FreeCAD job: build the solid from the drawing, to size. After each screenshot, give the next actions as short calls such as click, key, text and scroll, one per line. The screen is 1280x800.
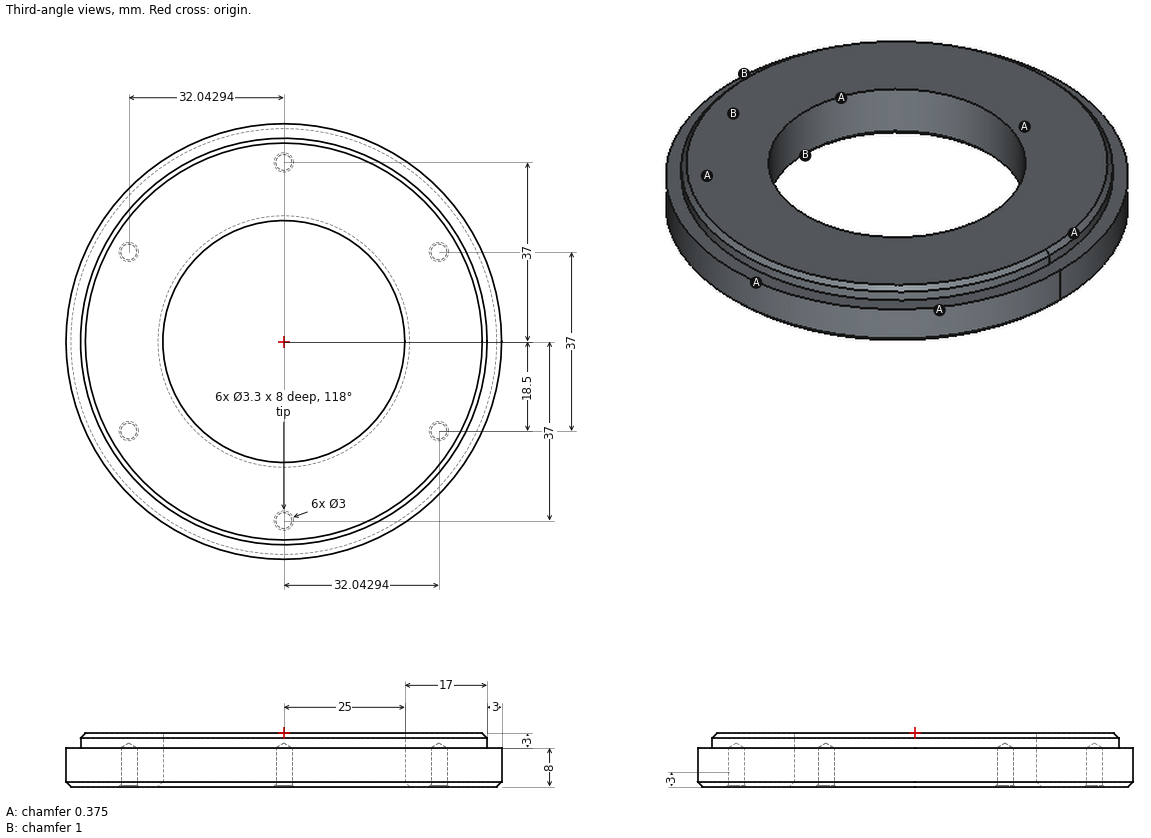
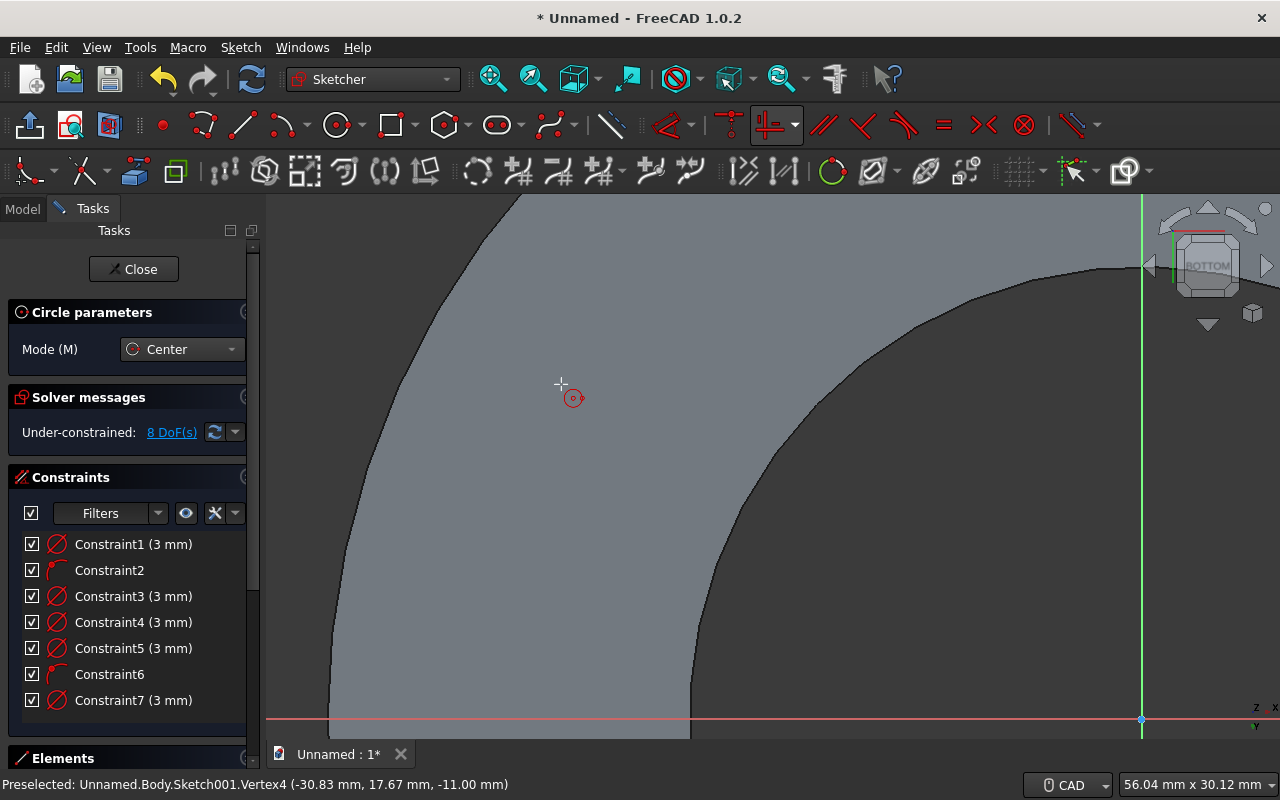
click(562, 385)
move(581, 366)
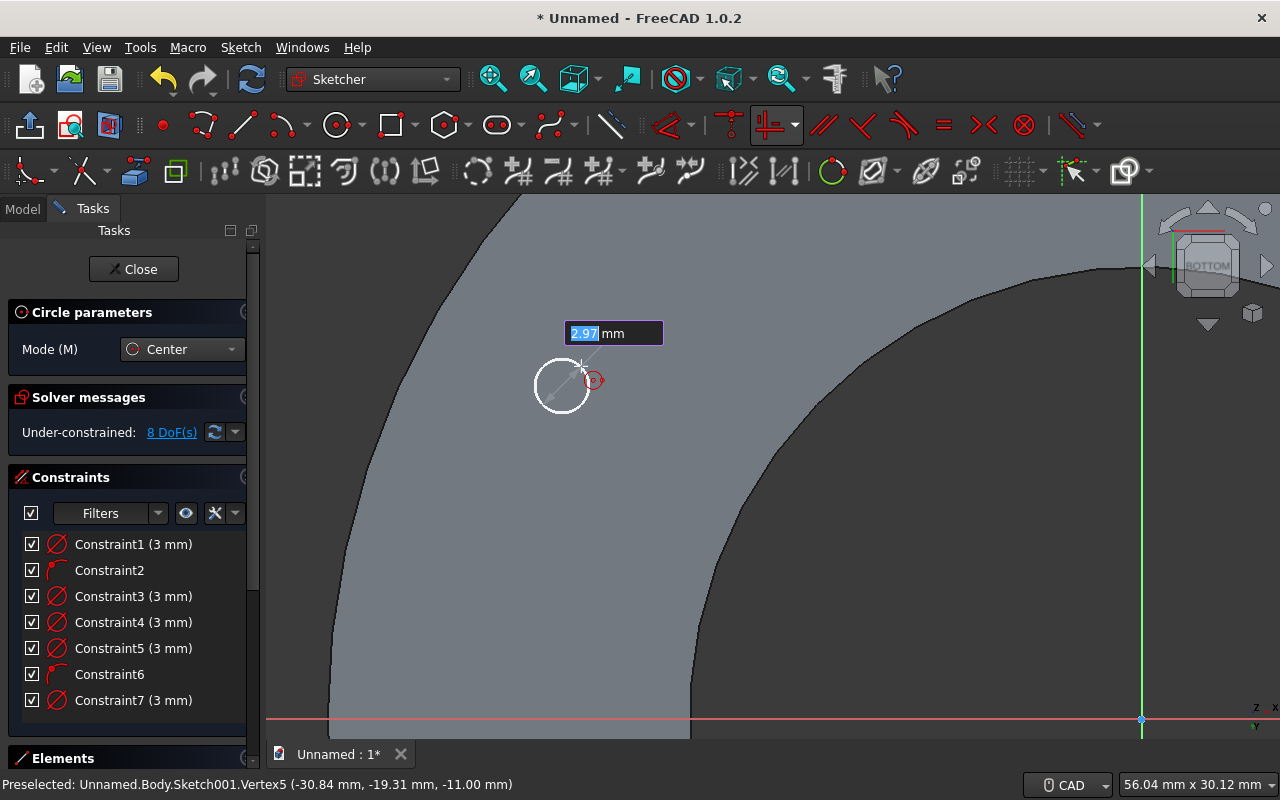
text(3)
key(Return)
key(Escape)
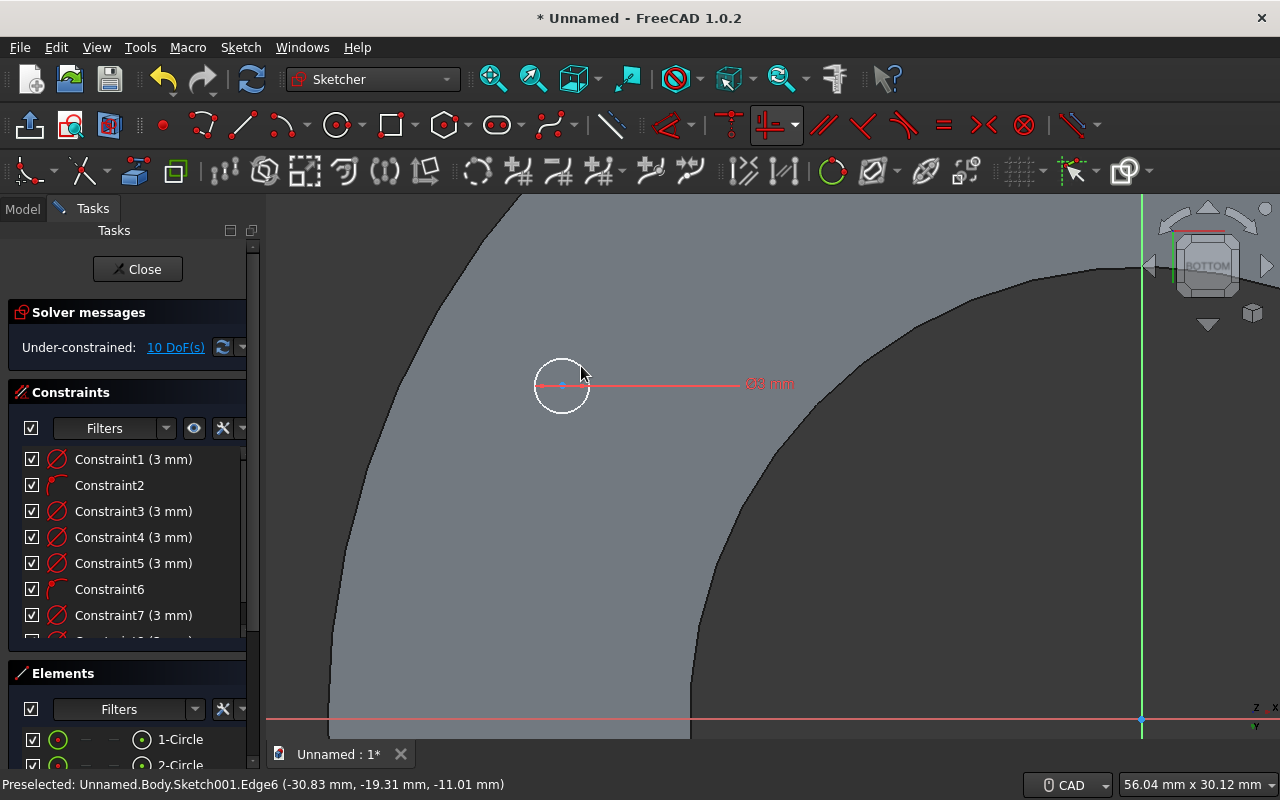
scroll(561, 384, down, 7)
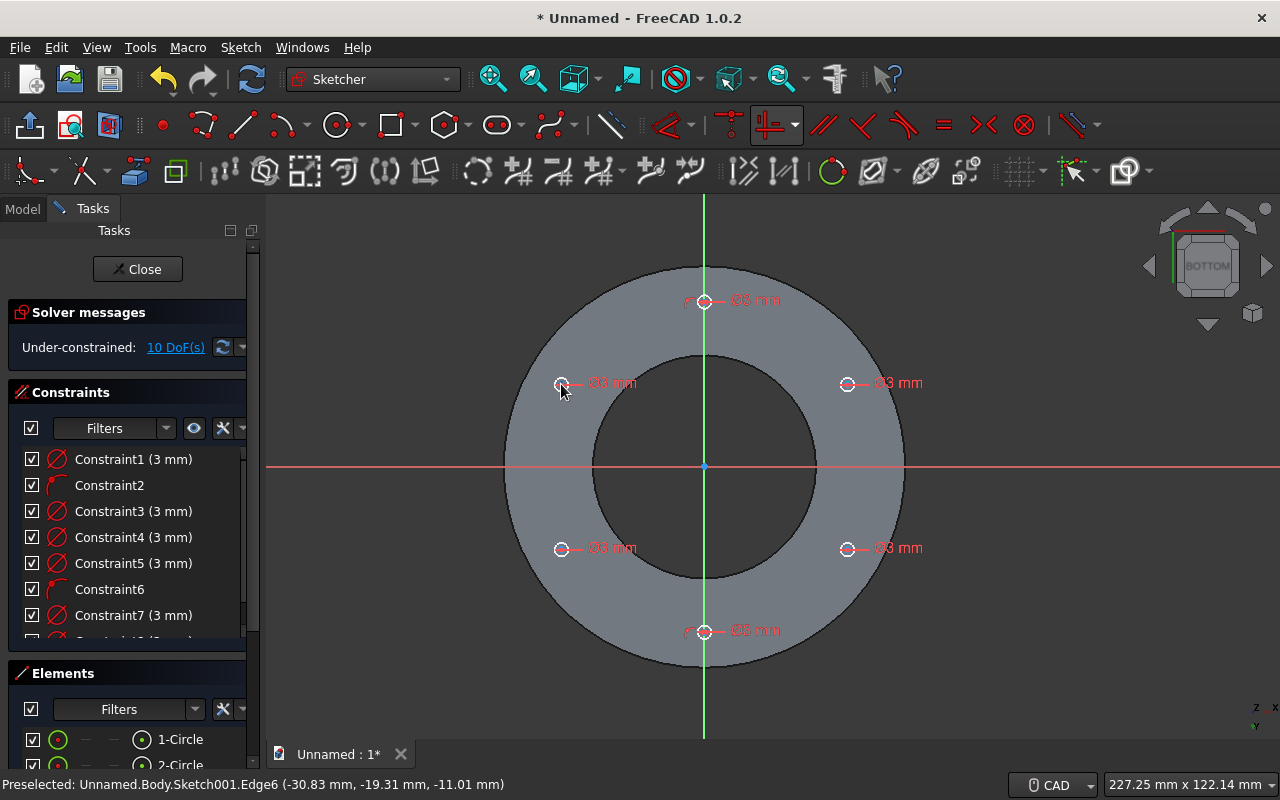
click(847, 385)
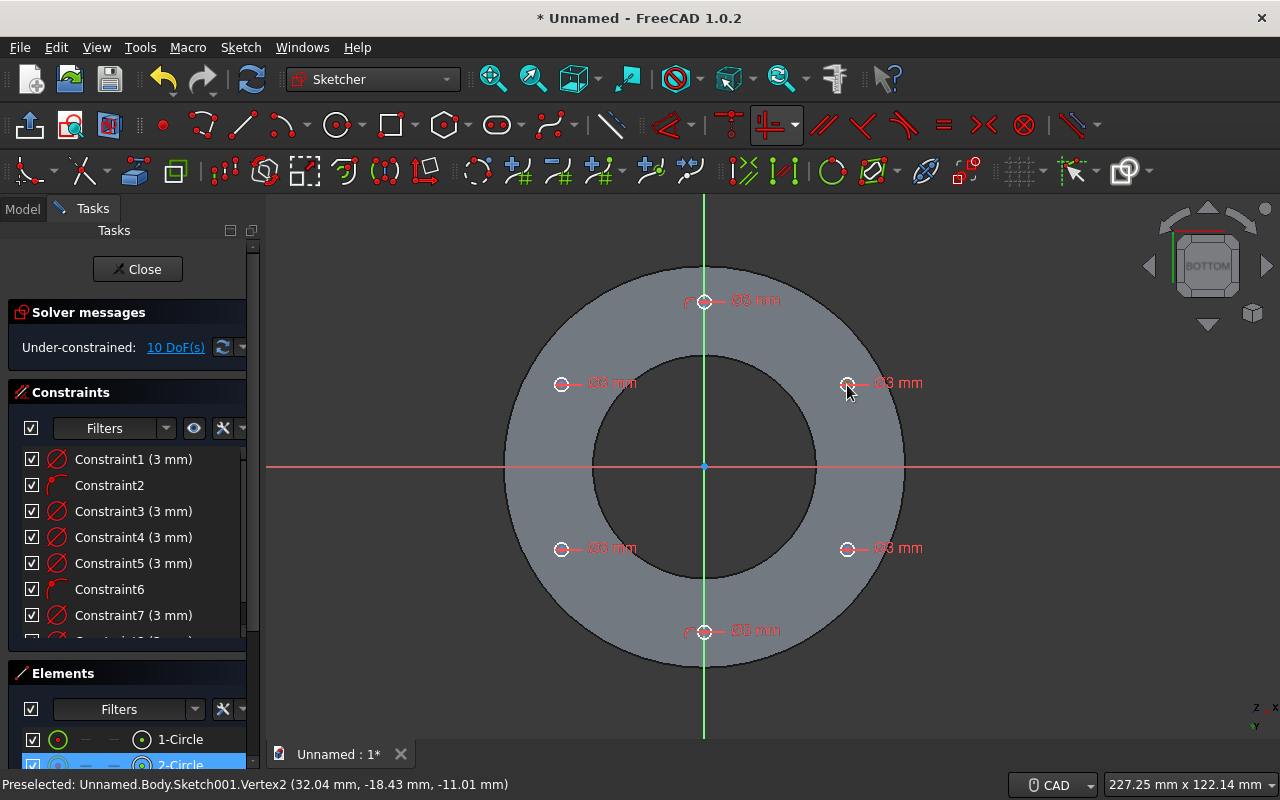
click(847, 550)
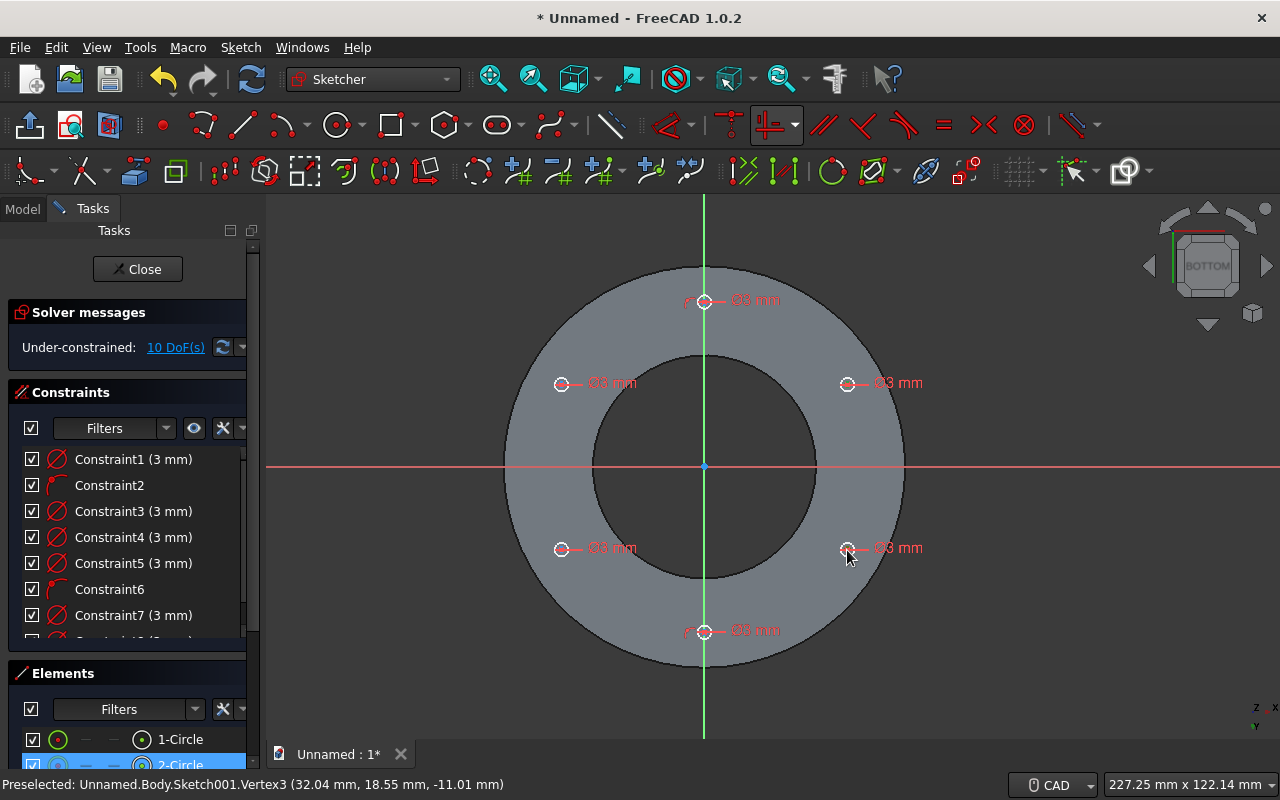
click(798, 126)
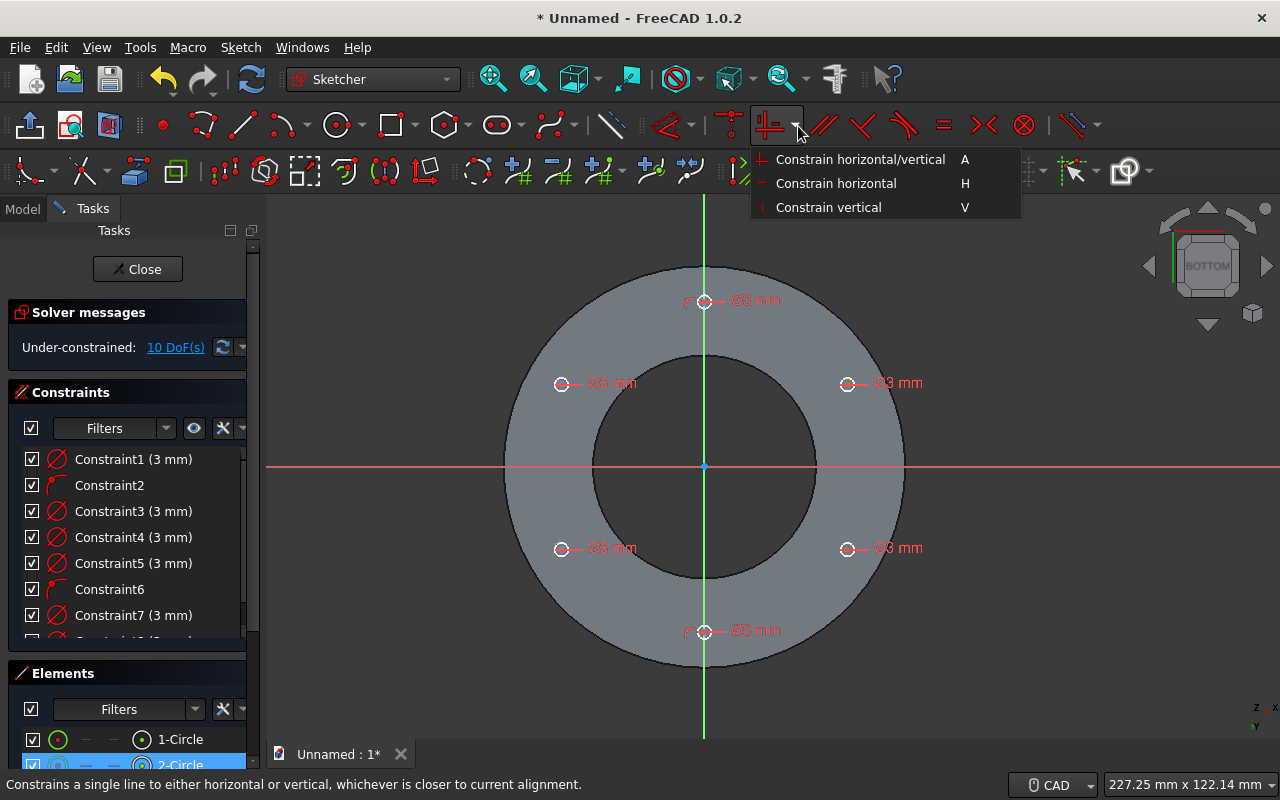
click(886, 207)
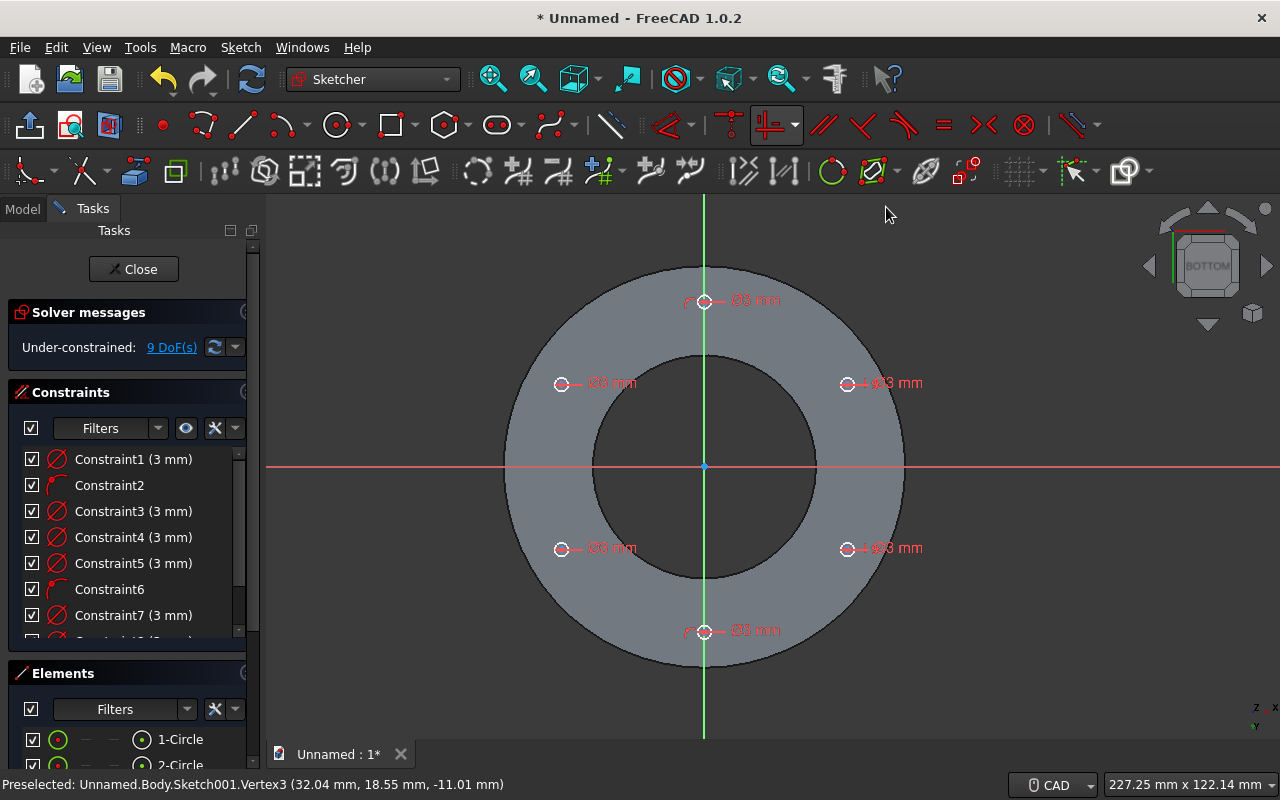
click(847, 550)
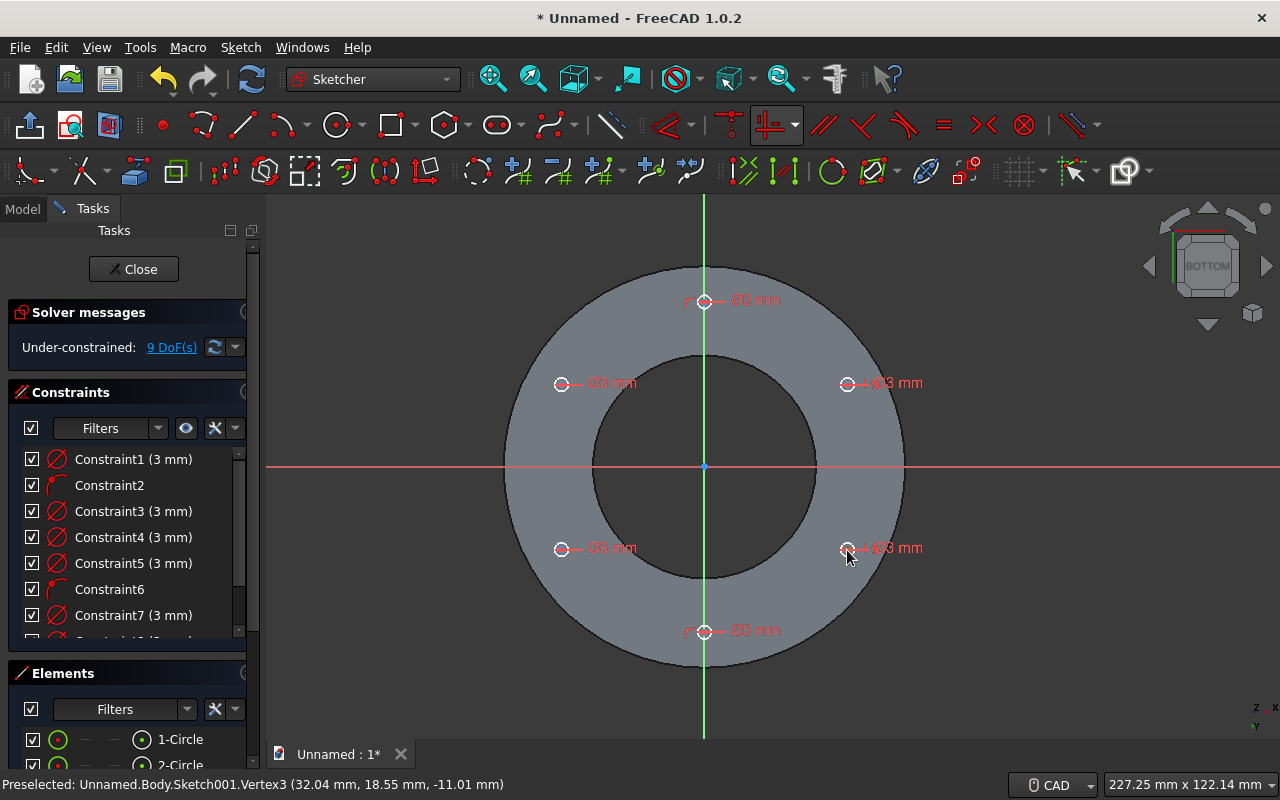
click(561, 550)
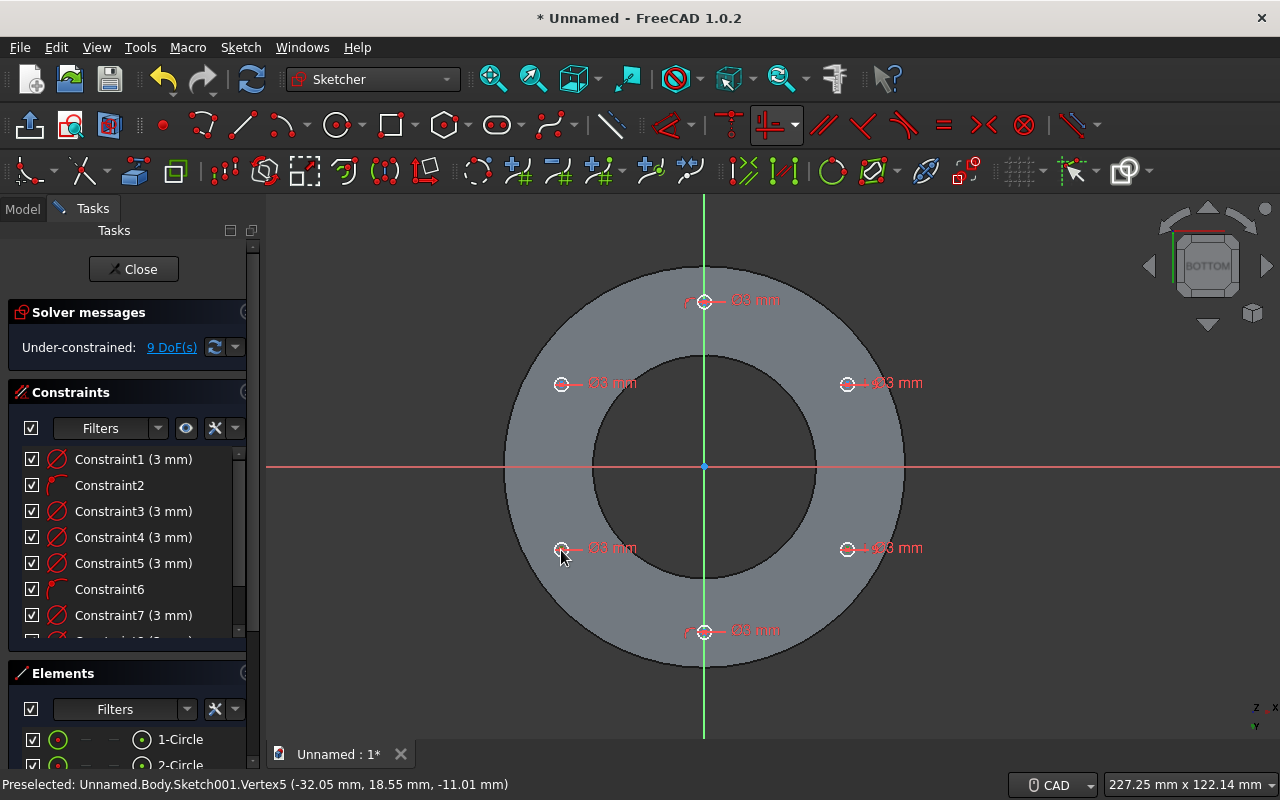
click(798, 126)